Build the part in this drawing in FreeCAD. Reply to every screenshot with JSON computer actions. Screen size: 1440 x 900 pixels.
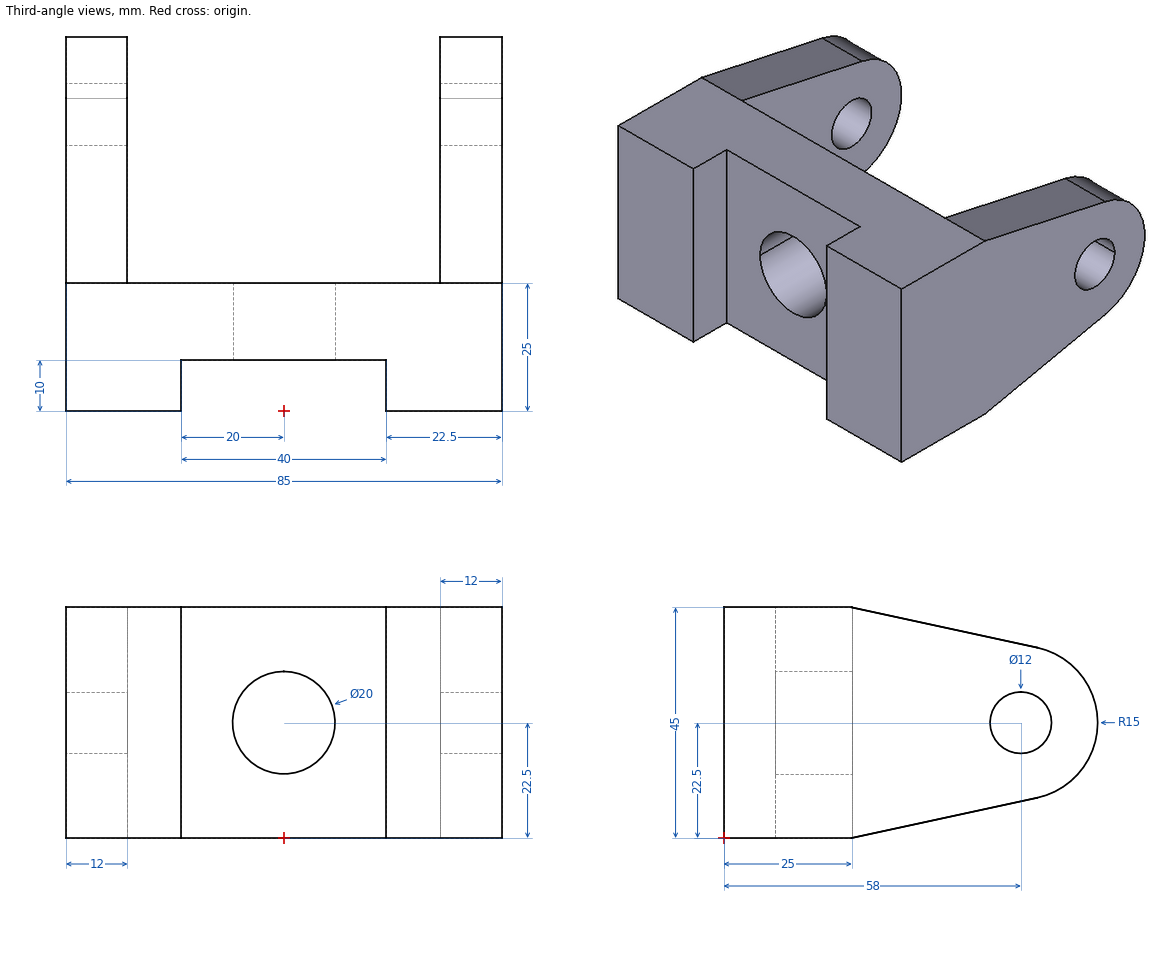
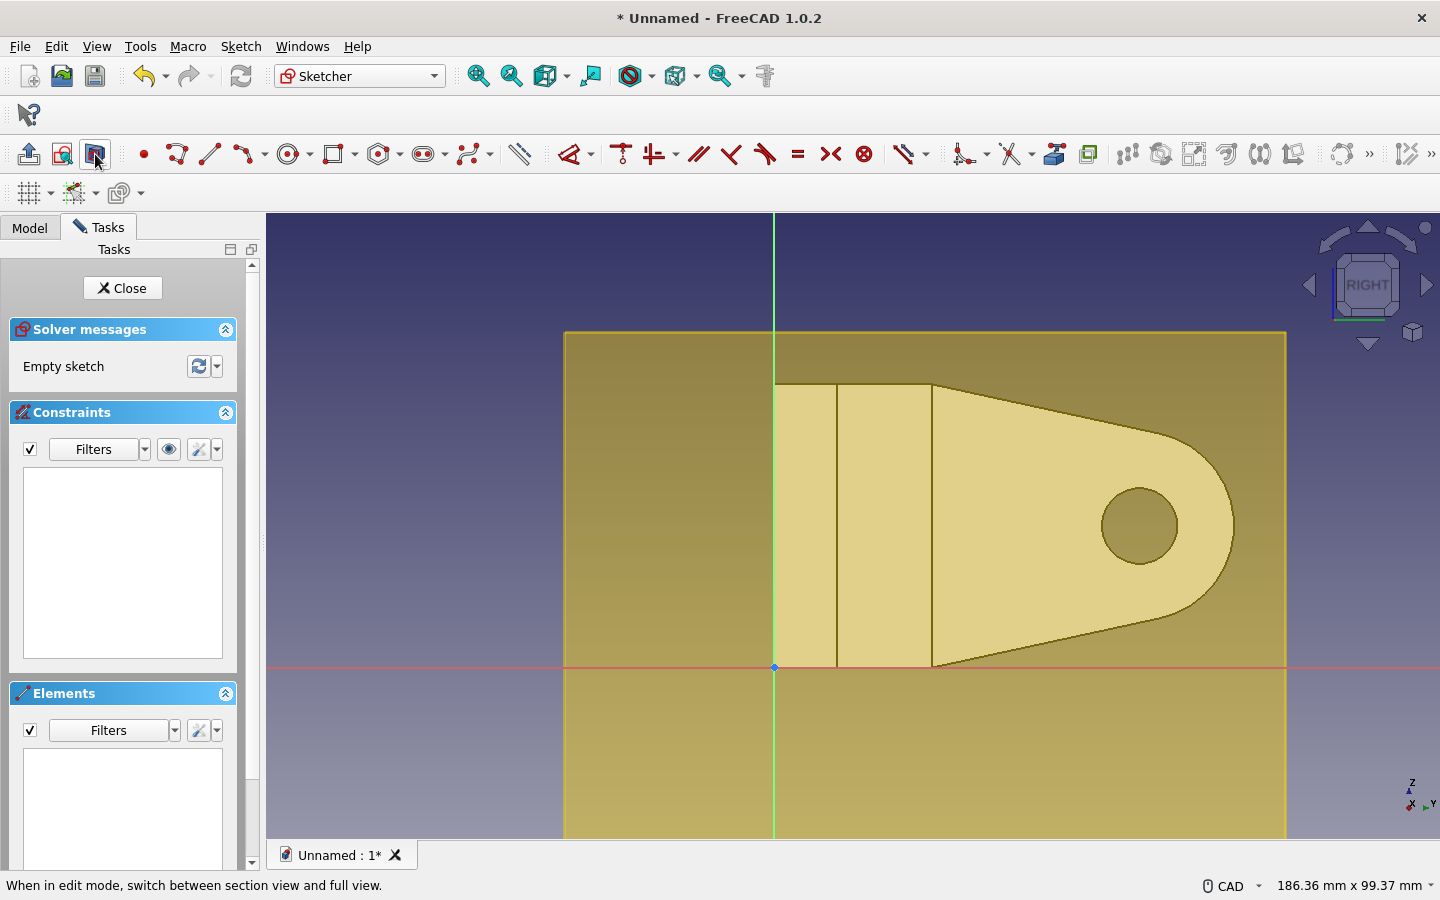
{"action": "scroll", "coordinate": [1275, 526], "scroll_direction": "up", "scroll_amount": 2}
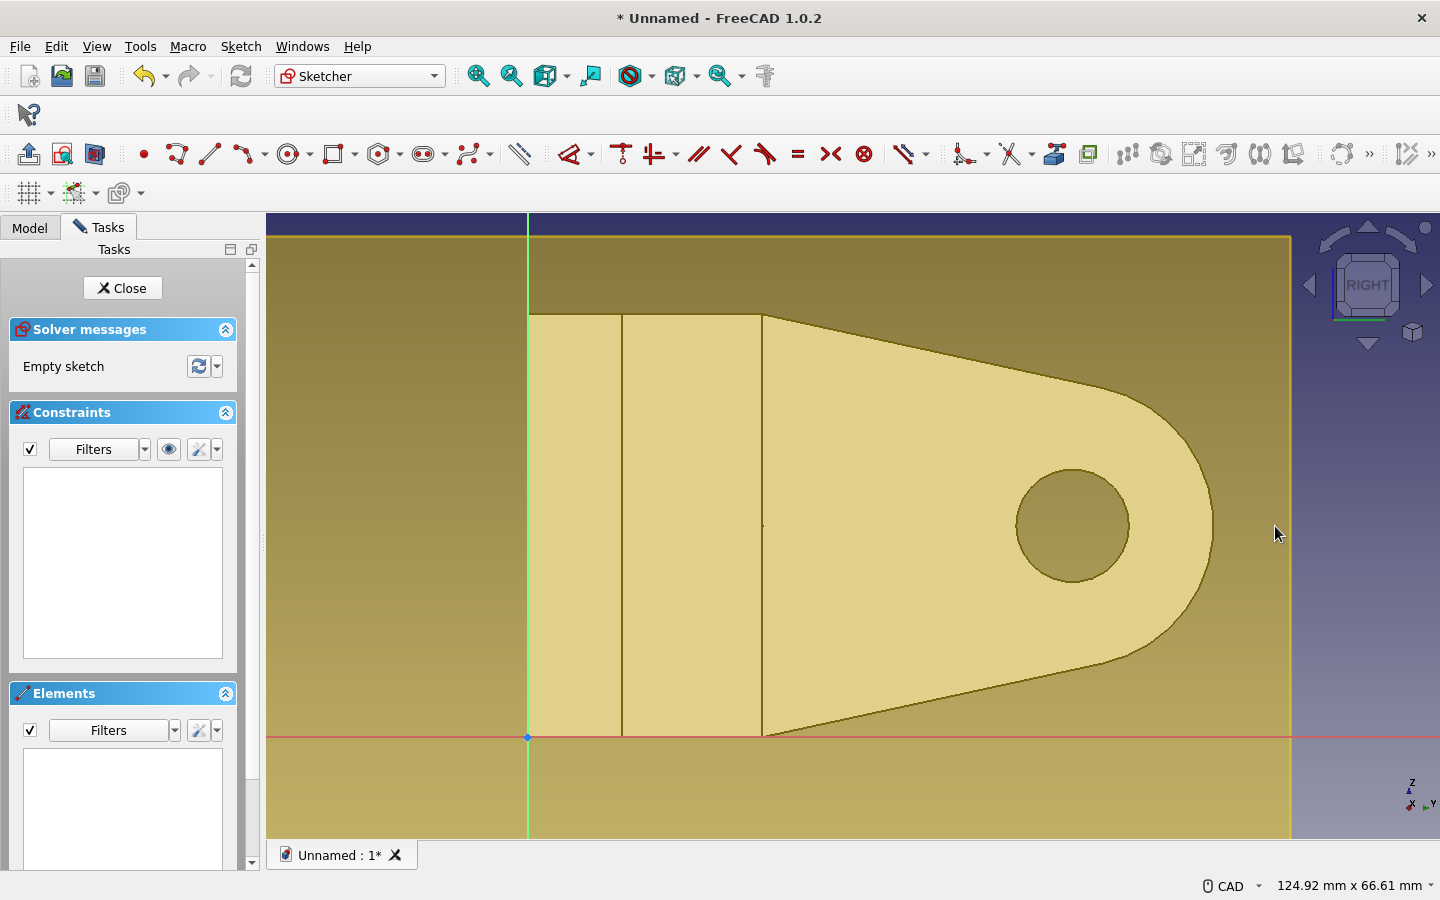
{"action": "left_click", "coordinate": [177, 154]}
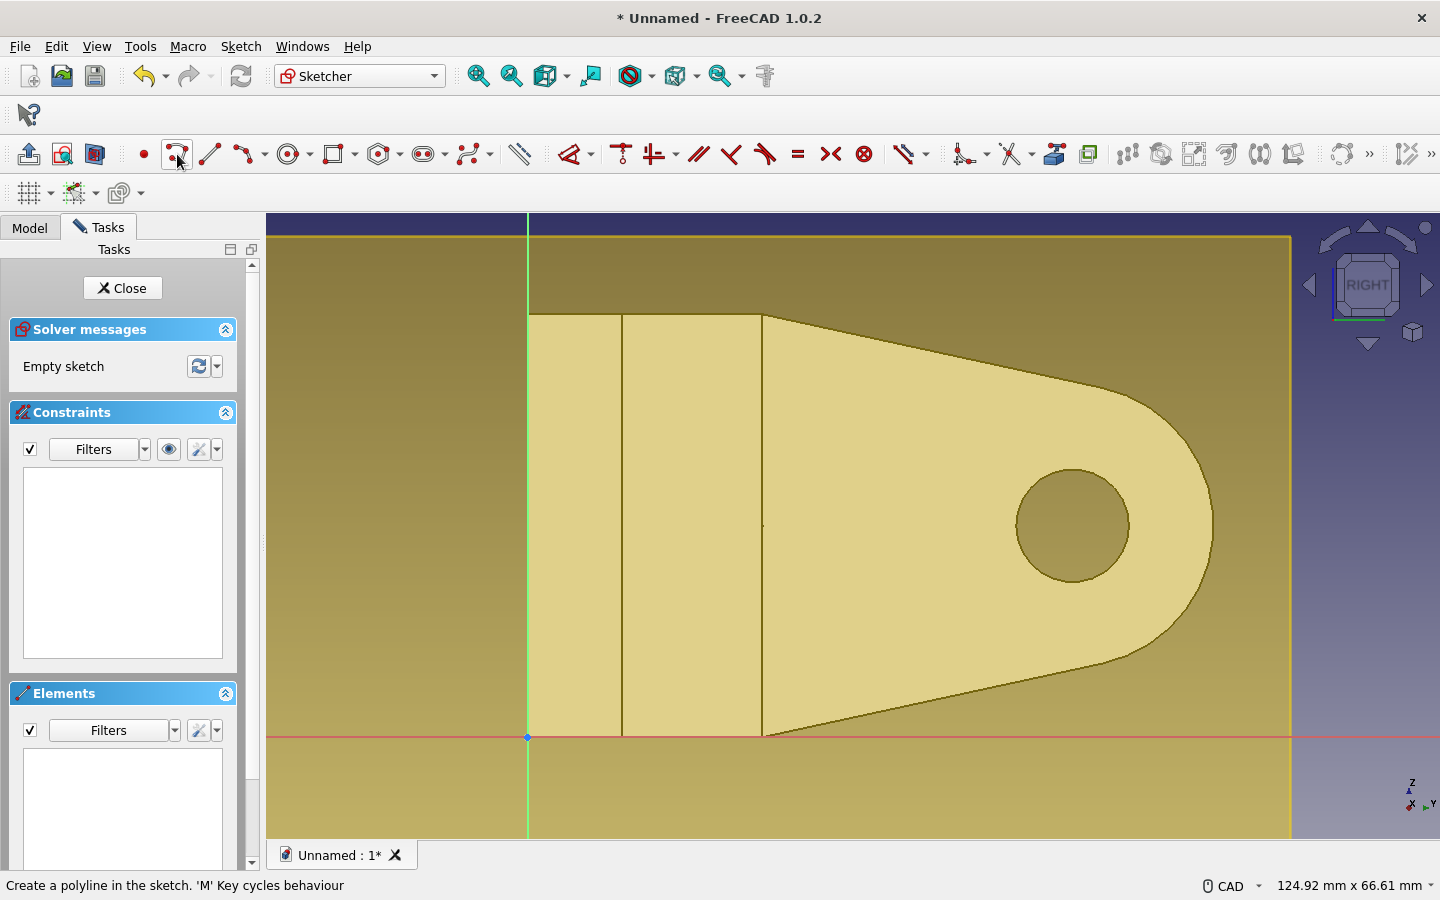
{"action": "left_click", "coordinate": [1102, 388]}
{"action": "left_click", "coordinate": [762, 314]}
{"action": "left_click", "coordinate": [762, 737]}
{"action": "left_click", "coordinate": [1102, 664]}
{"action": "right_click", "coordinate": [1102, 664]}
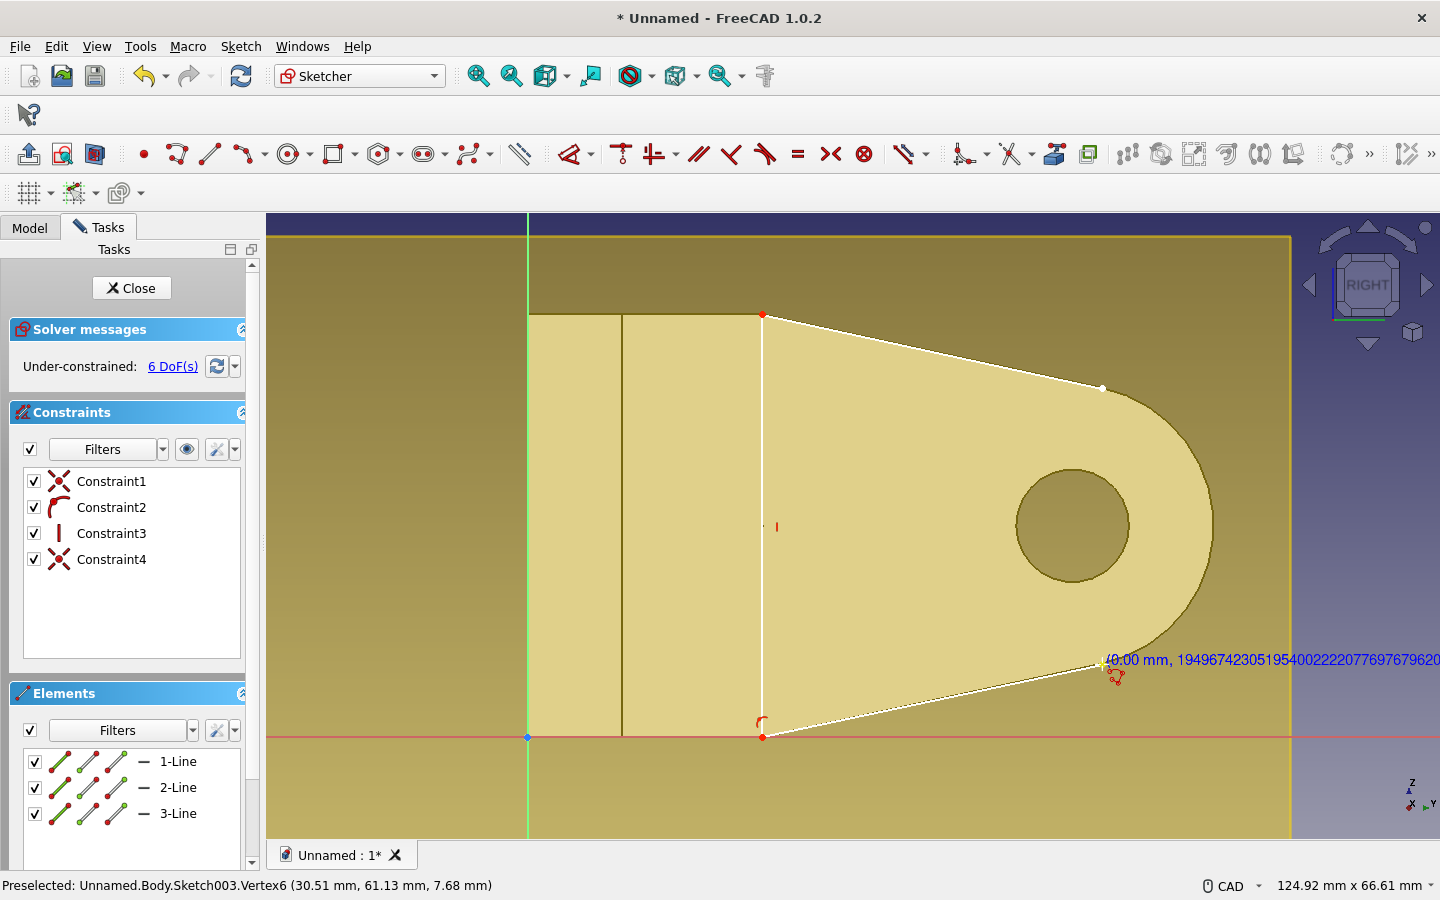
{"action": "left_click", "coordinate": [242, 154]}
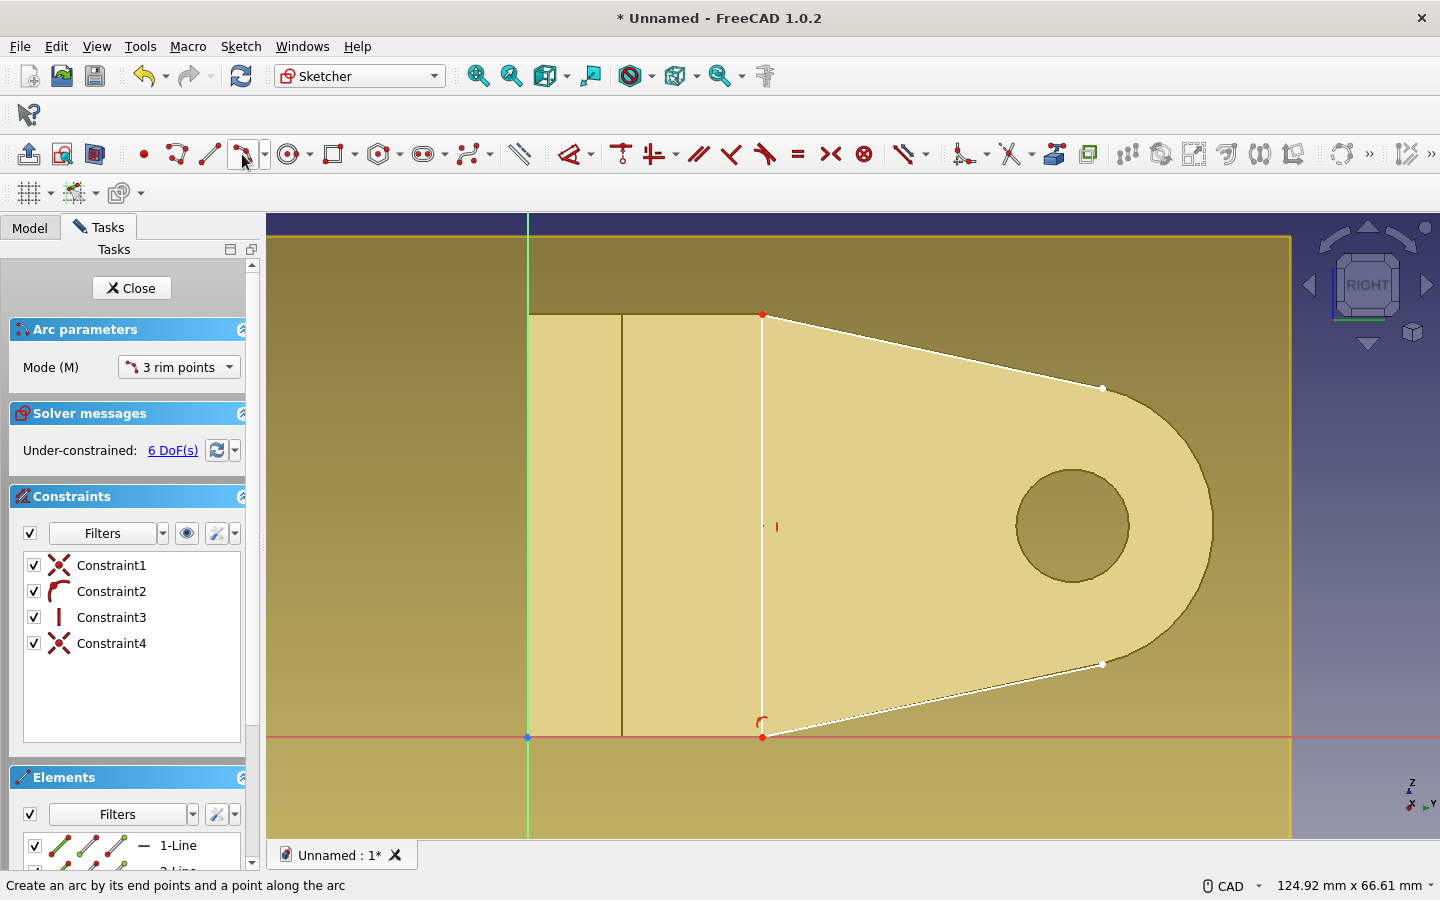
{"action": "left_click", "coordinate": [1102, 665]}
{"action": "left_click", "coordinate": [1102, 389]}
{"action": "left_click", "coordinate": [1214, 526]}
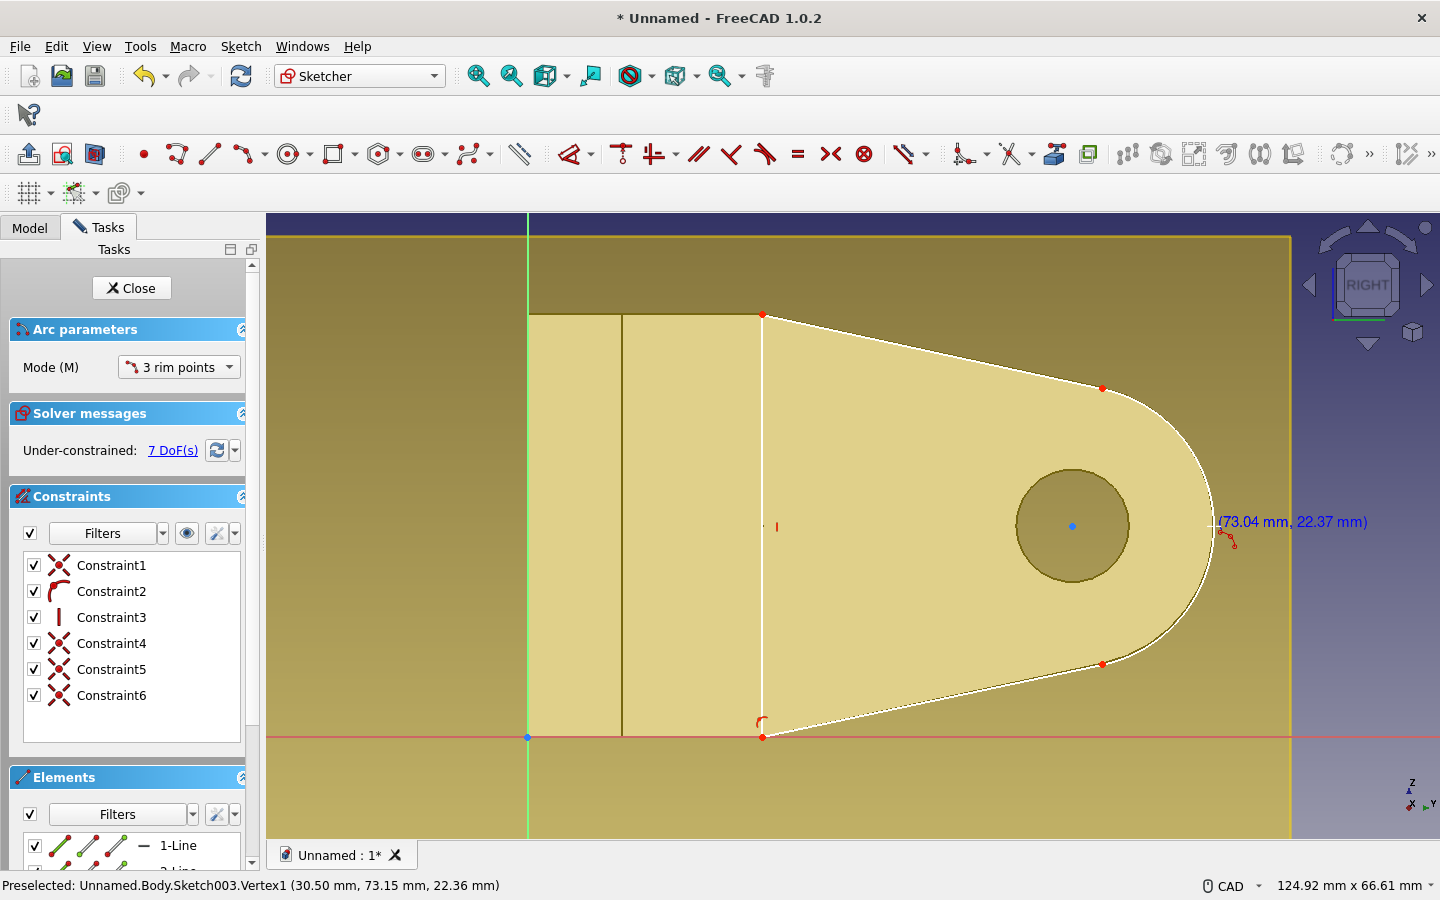
{"action": "left_click", "coordinate": [288, 154]}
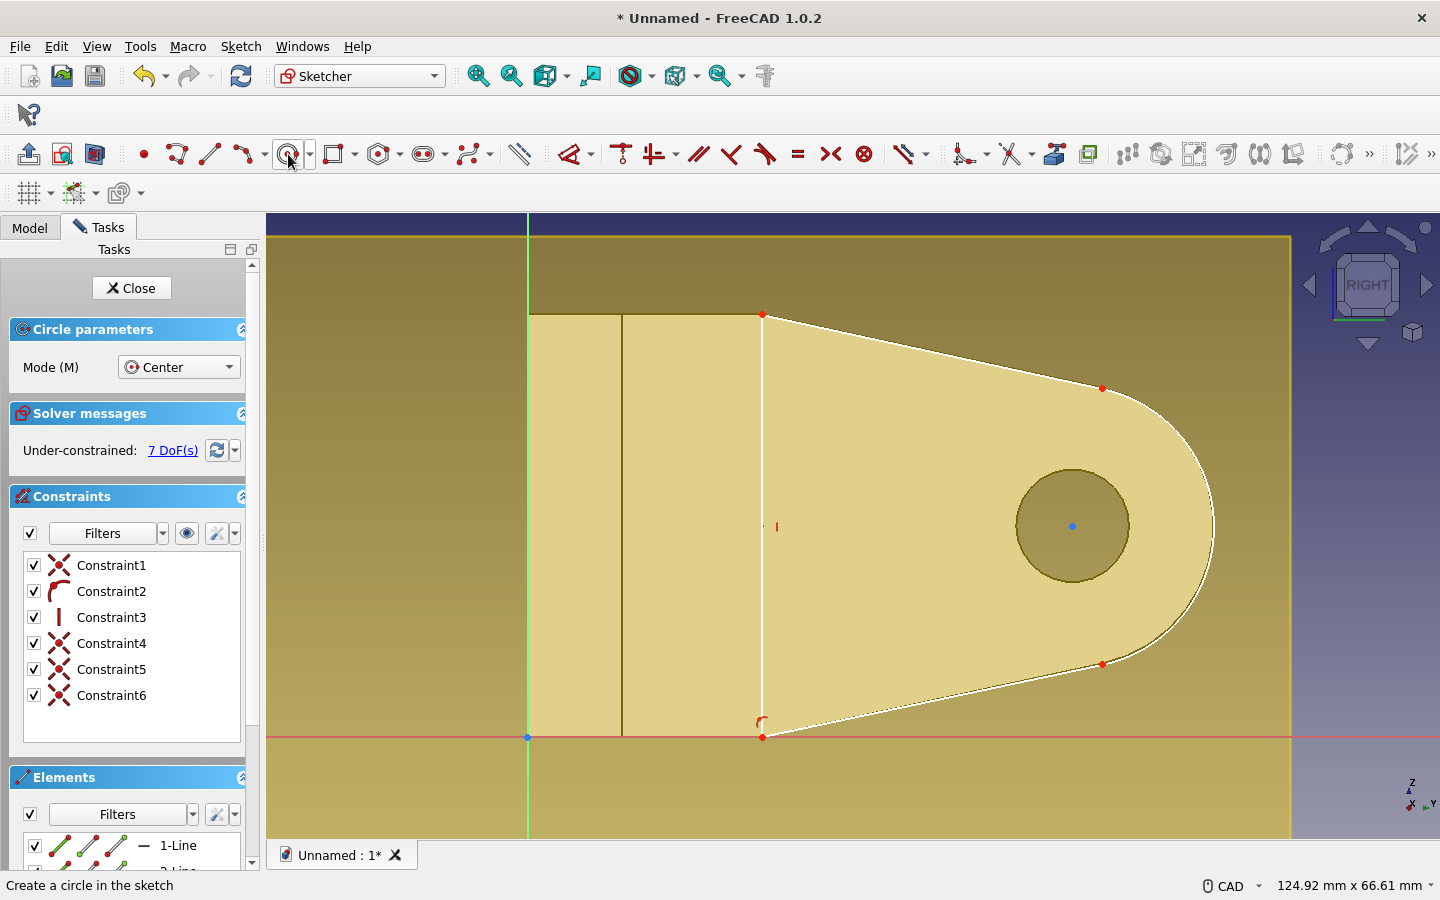
{"action": "left_click", "coordinate": [1073, 526]}
{"action": "mouse_move", "coordinate": [1112, 486]}